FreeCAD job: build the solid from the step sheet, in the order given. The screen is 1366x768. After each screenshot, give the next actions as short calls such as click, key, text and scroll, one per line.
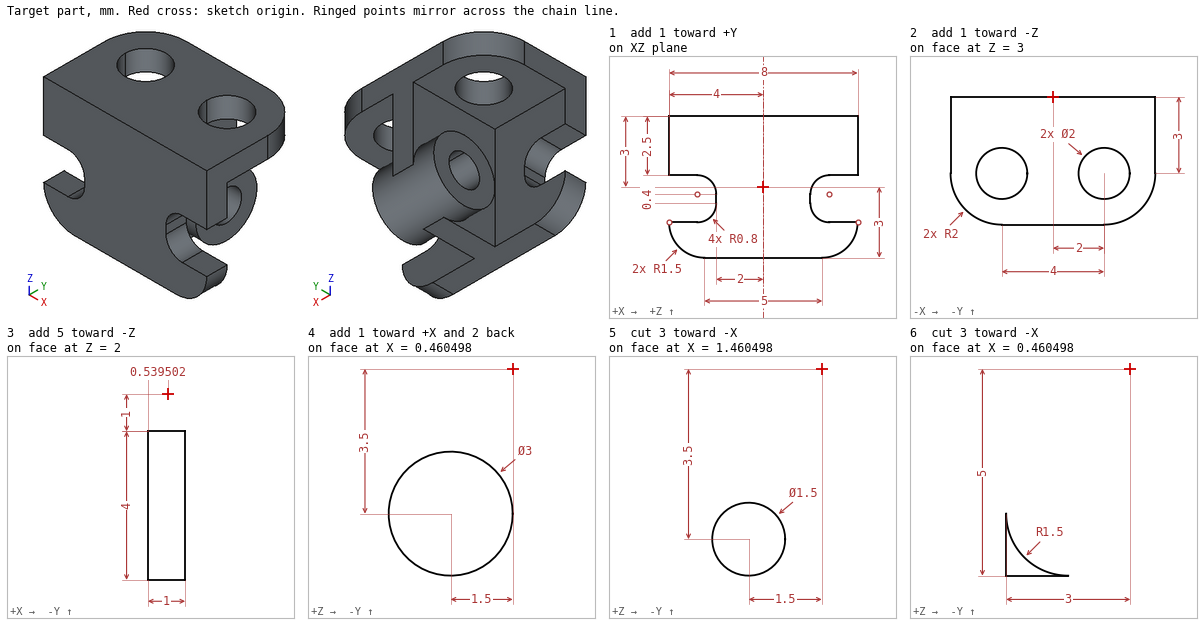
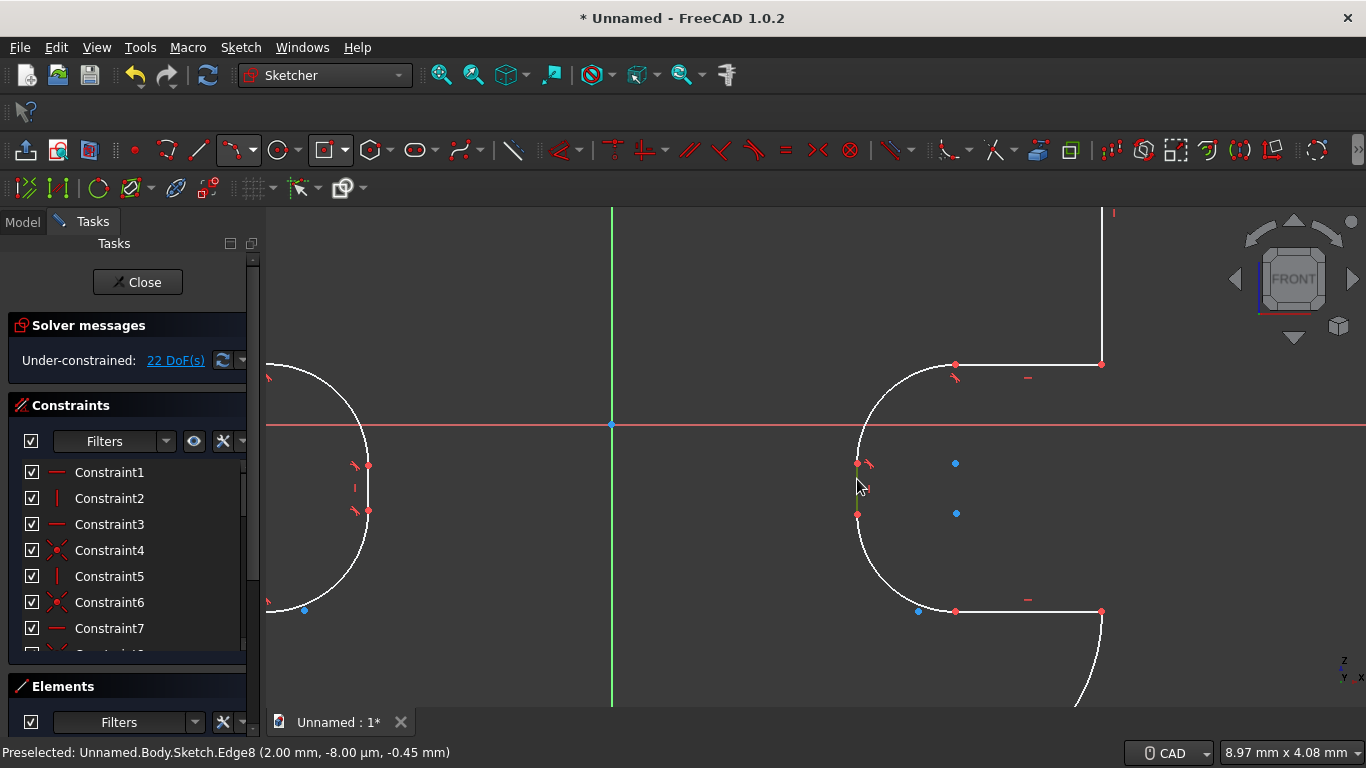
click(868, 558)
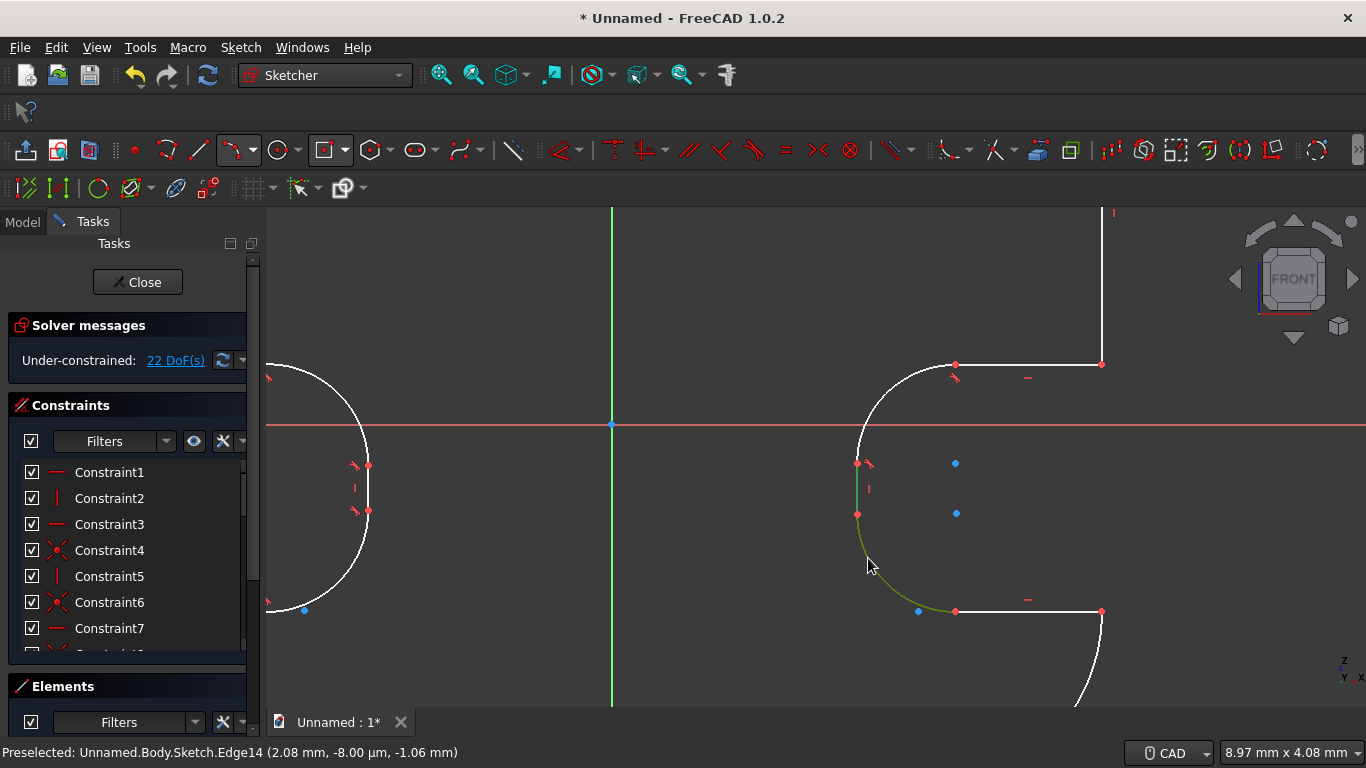
click(754, 150)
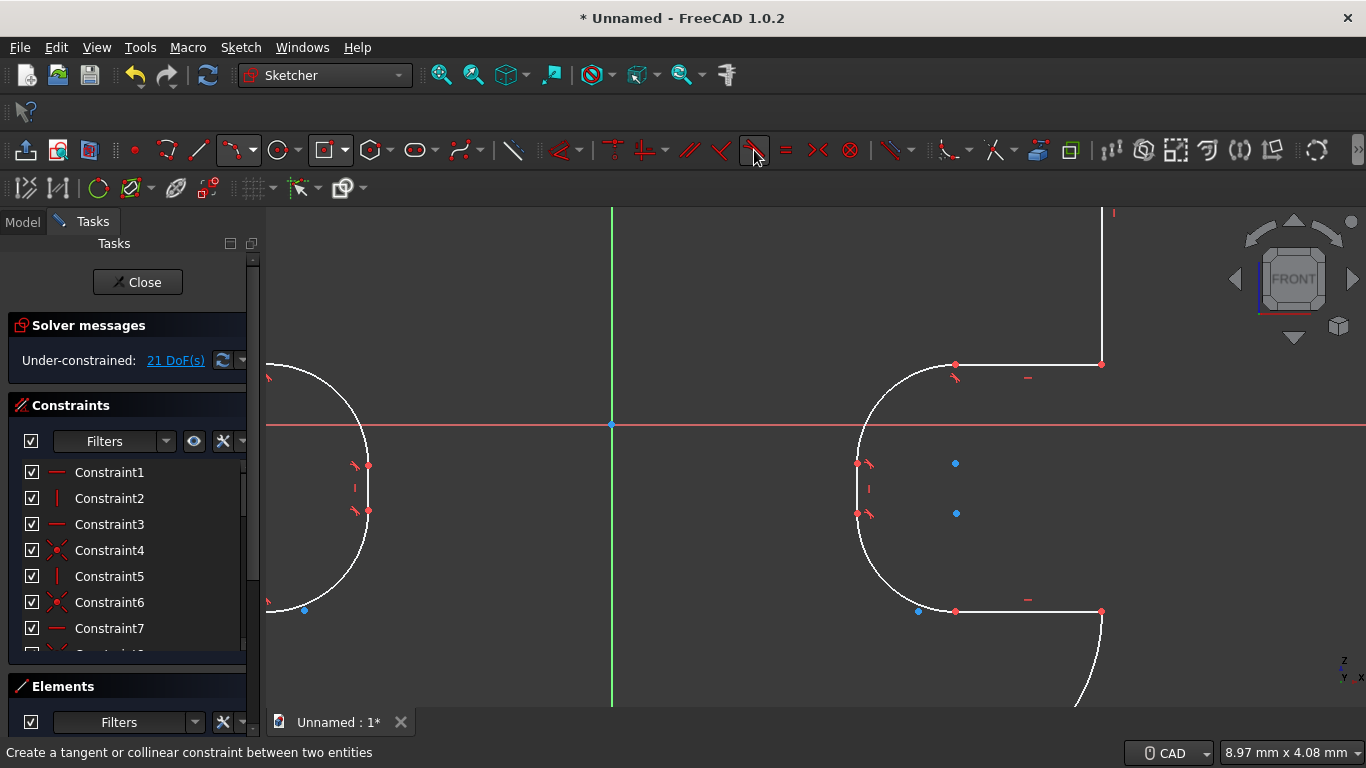
click(999, 612)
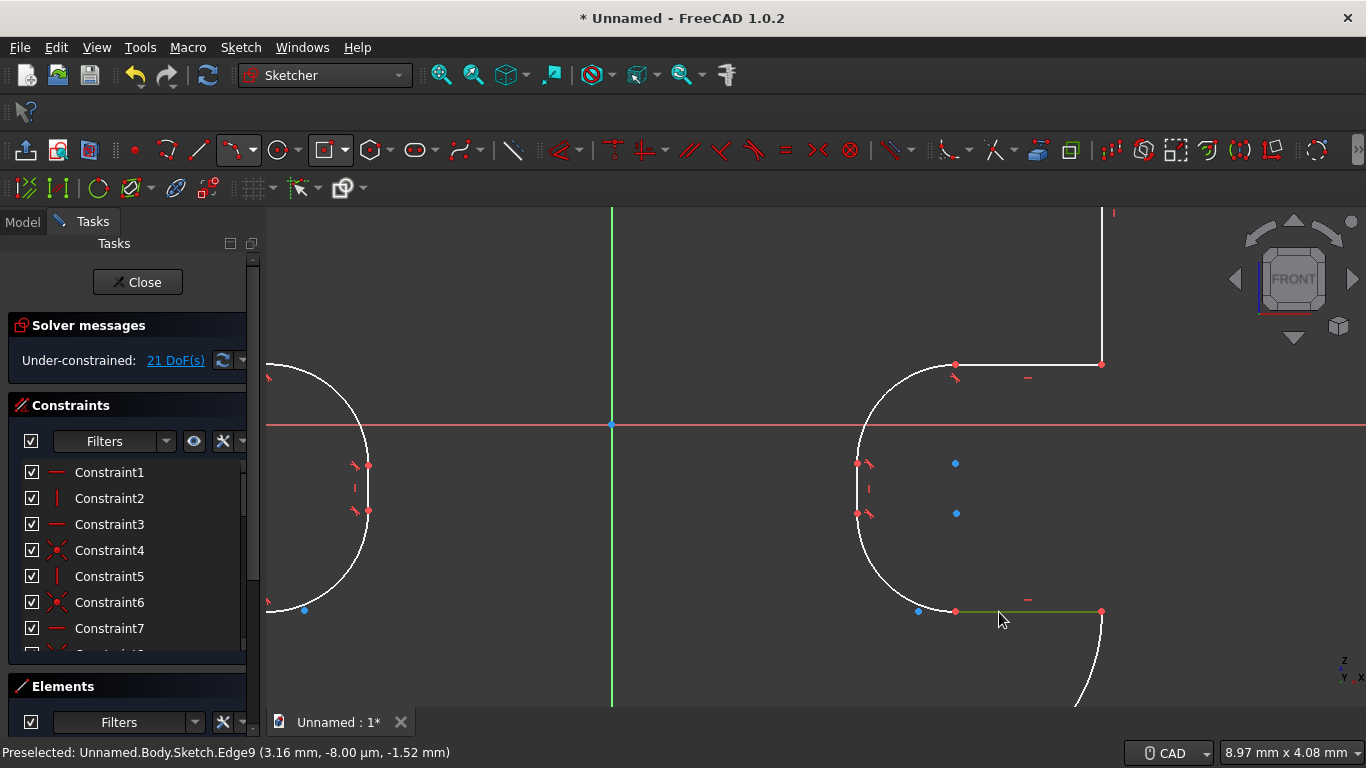
click(868, 558)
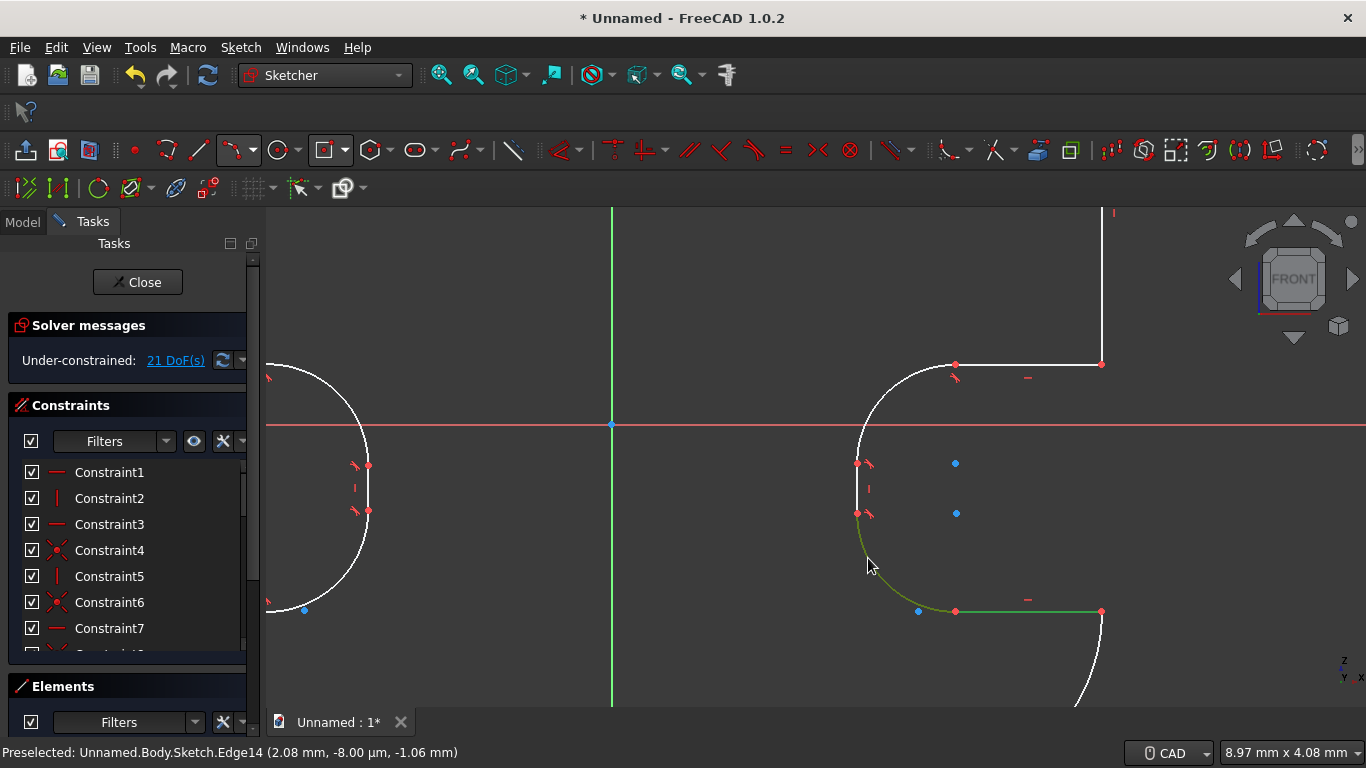
click(754, 150)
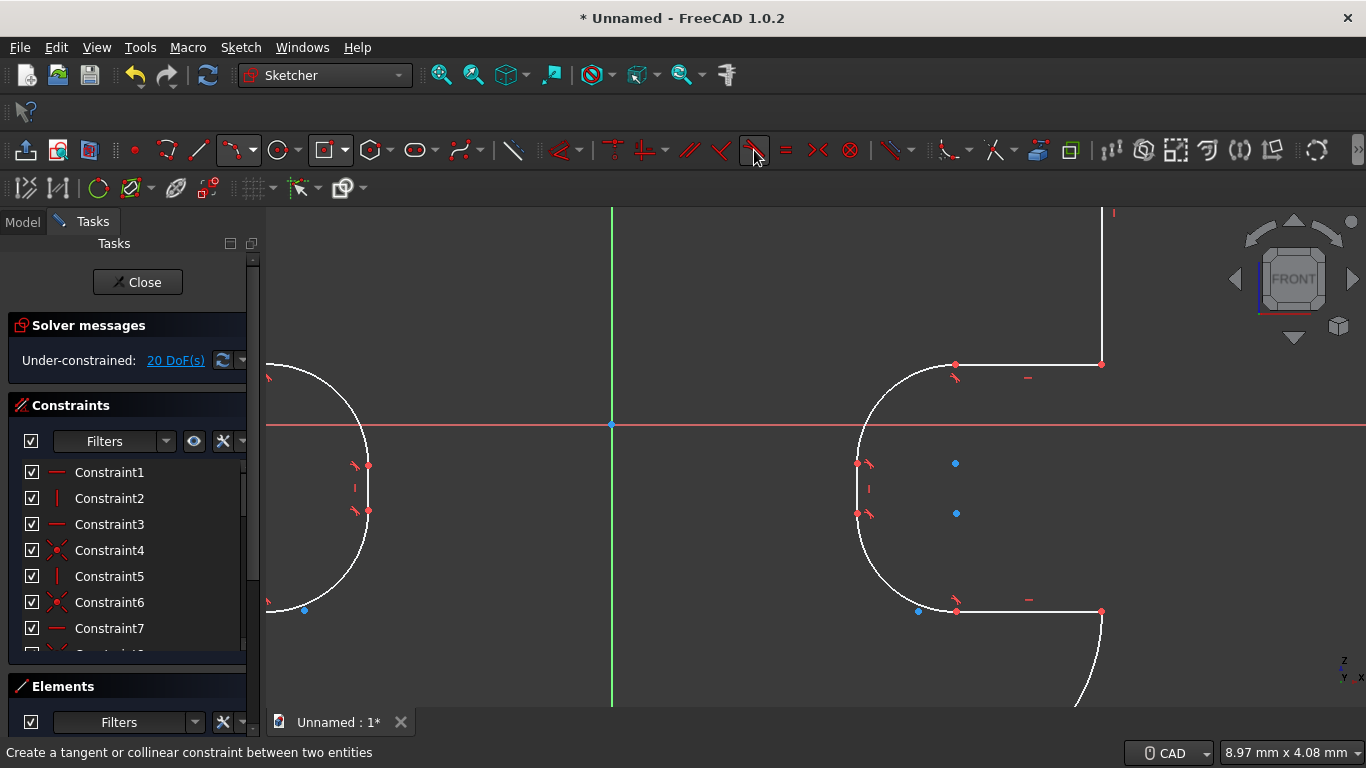
scroll(858, 483, down, 4)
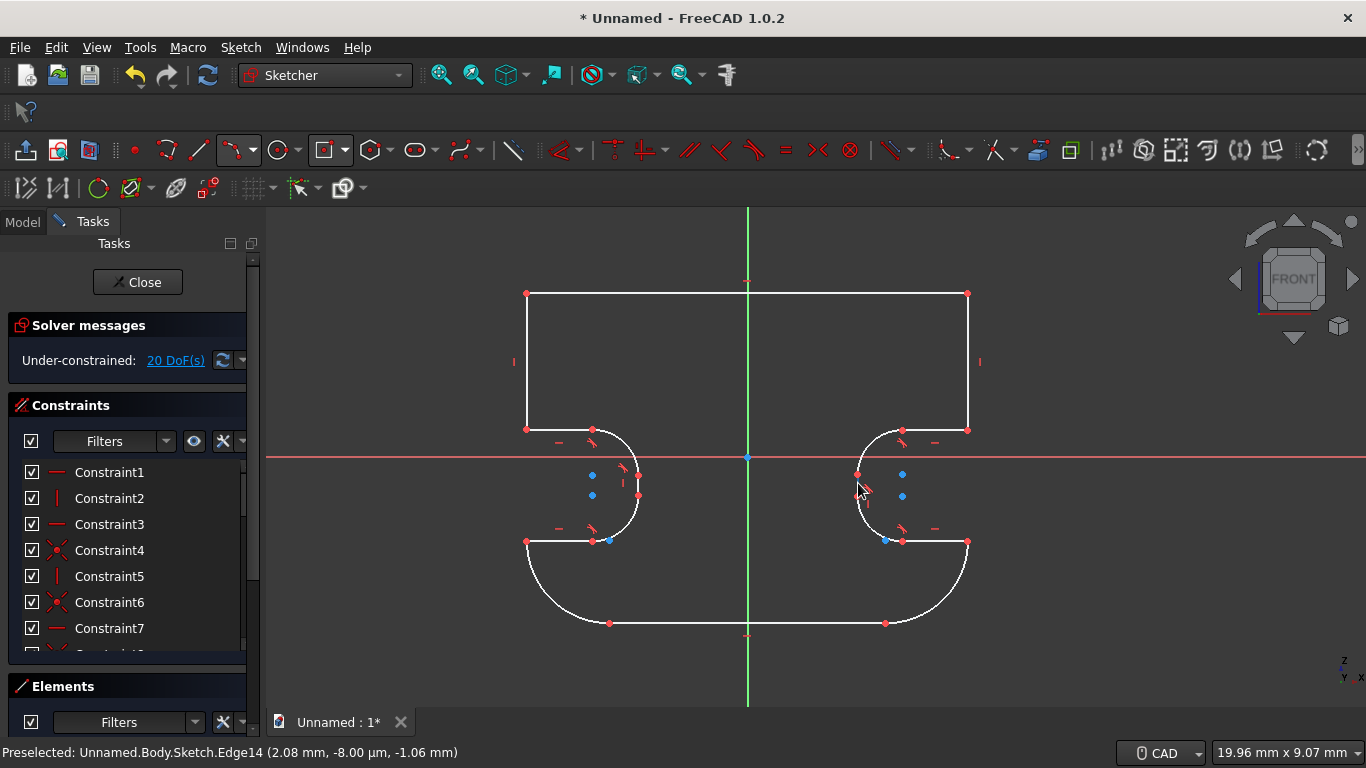
click(803, 623)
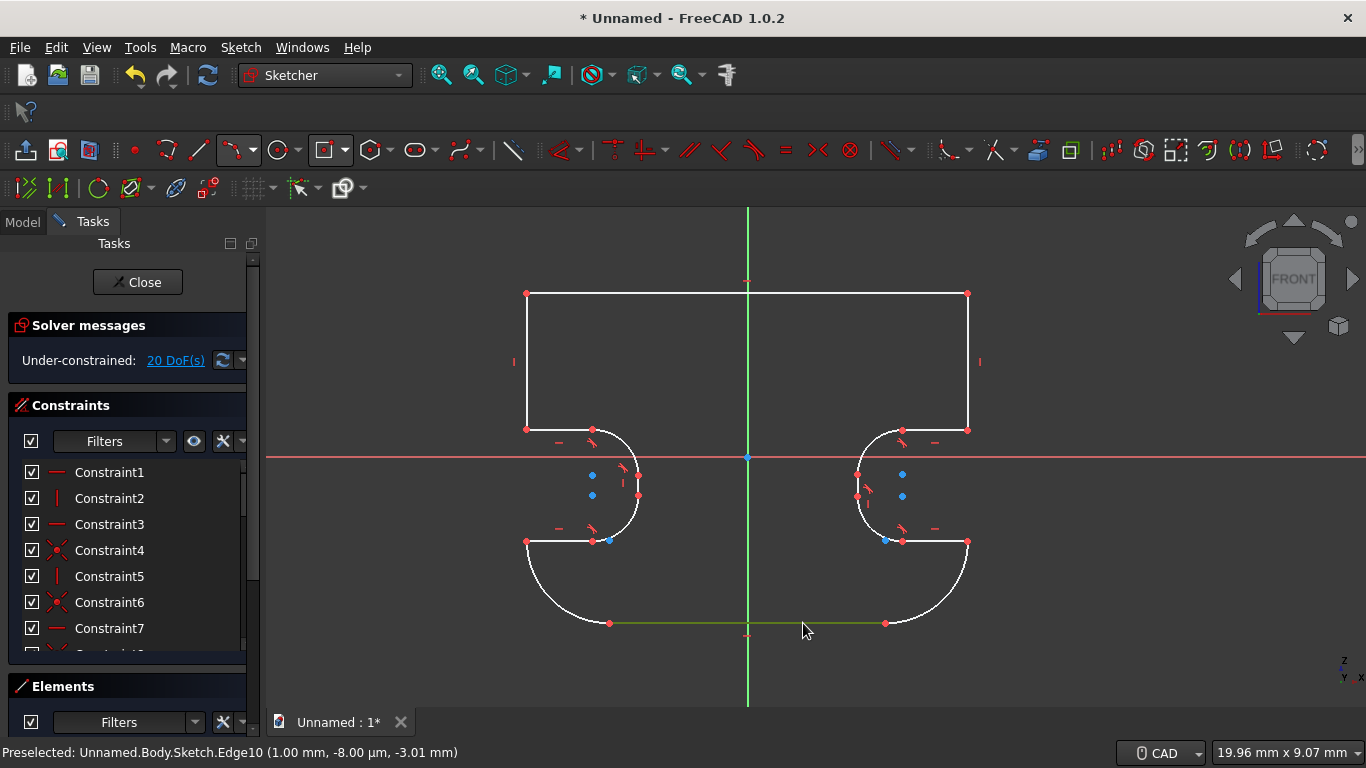
click(923, 614)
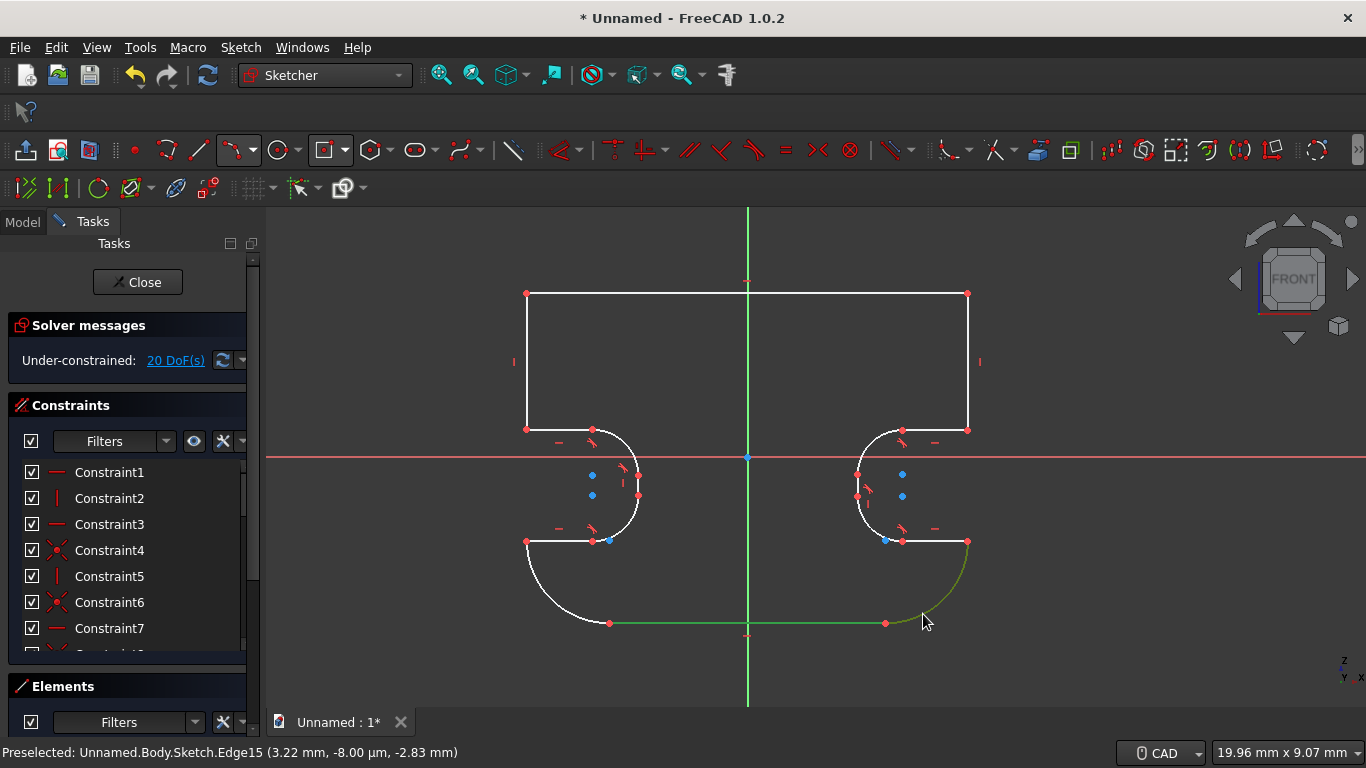
click(754, 150)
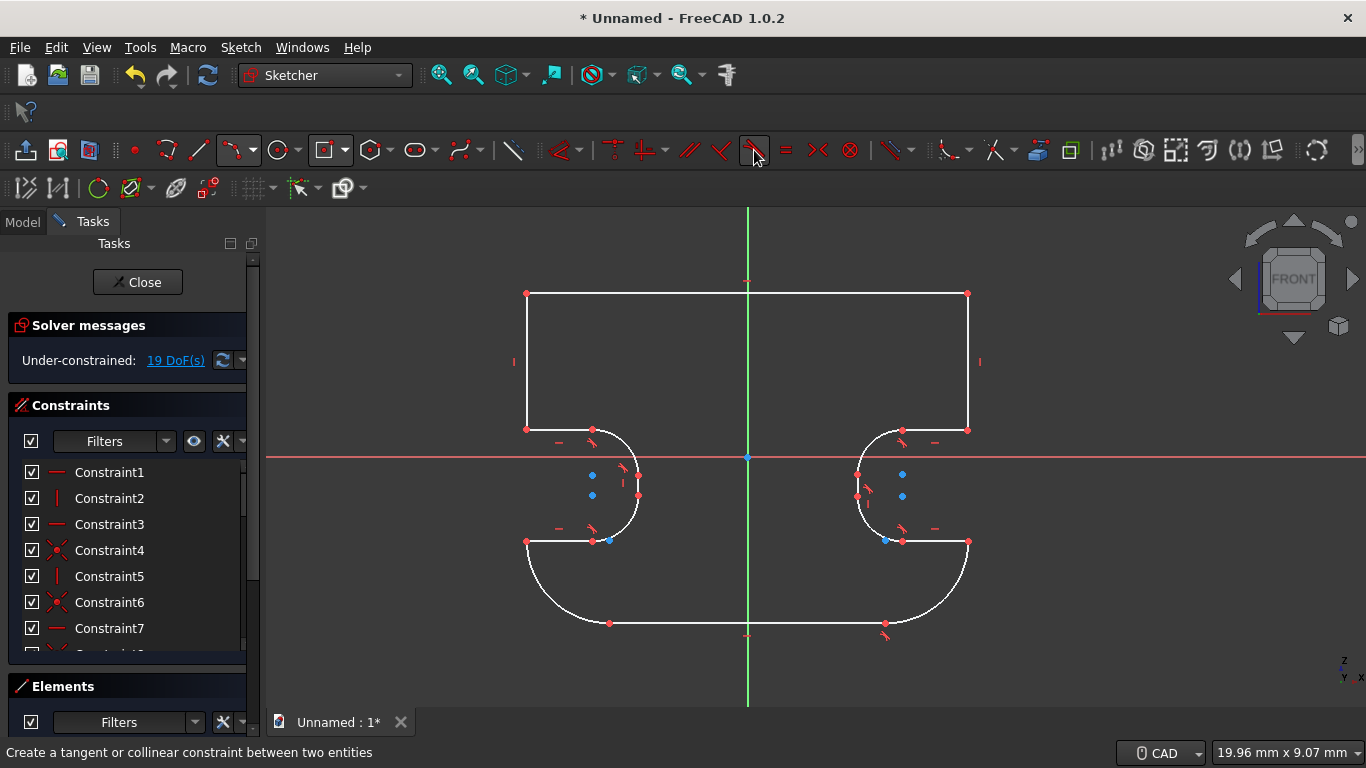
click(803, 623)